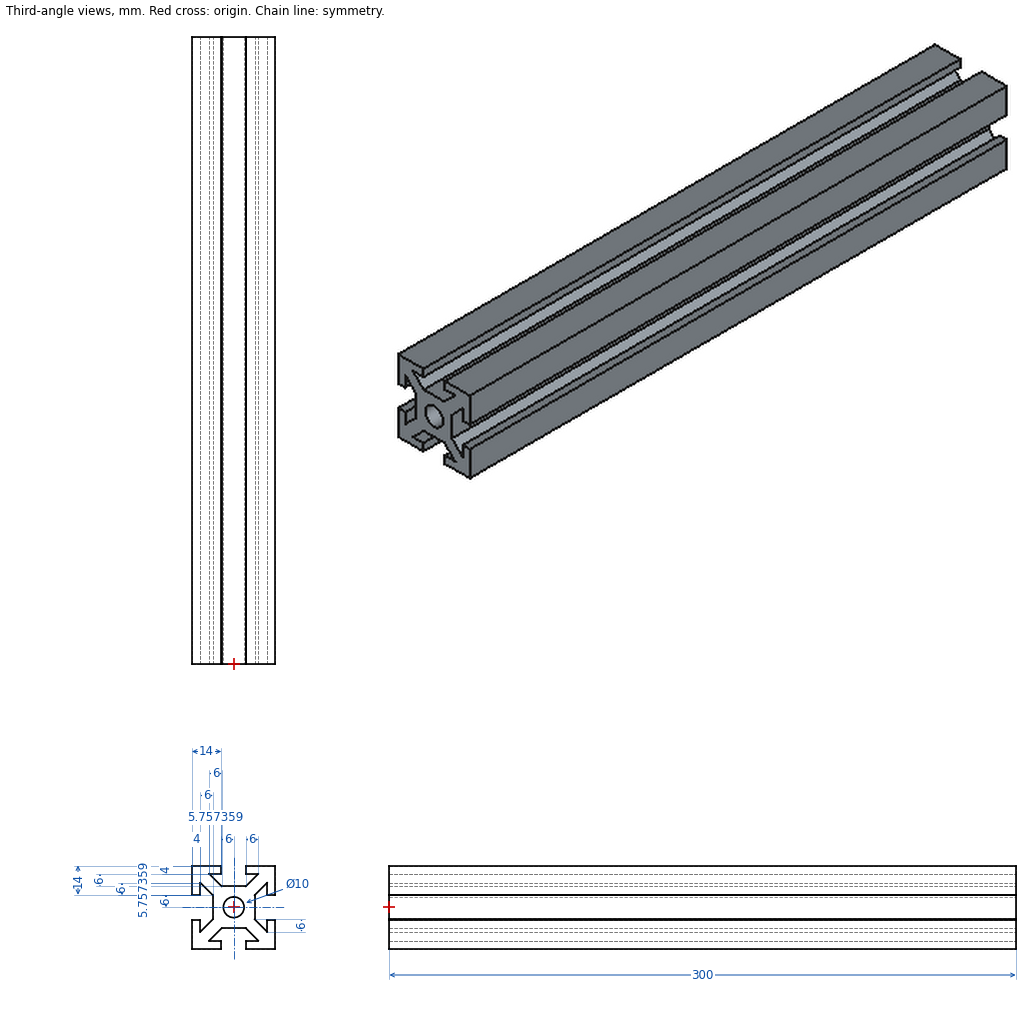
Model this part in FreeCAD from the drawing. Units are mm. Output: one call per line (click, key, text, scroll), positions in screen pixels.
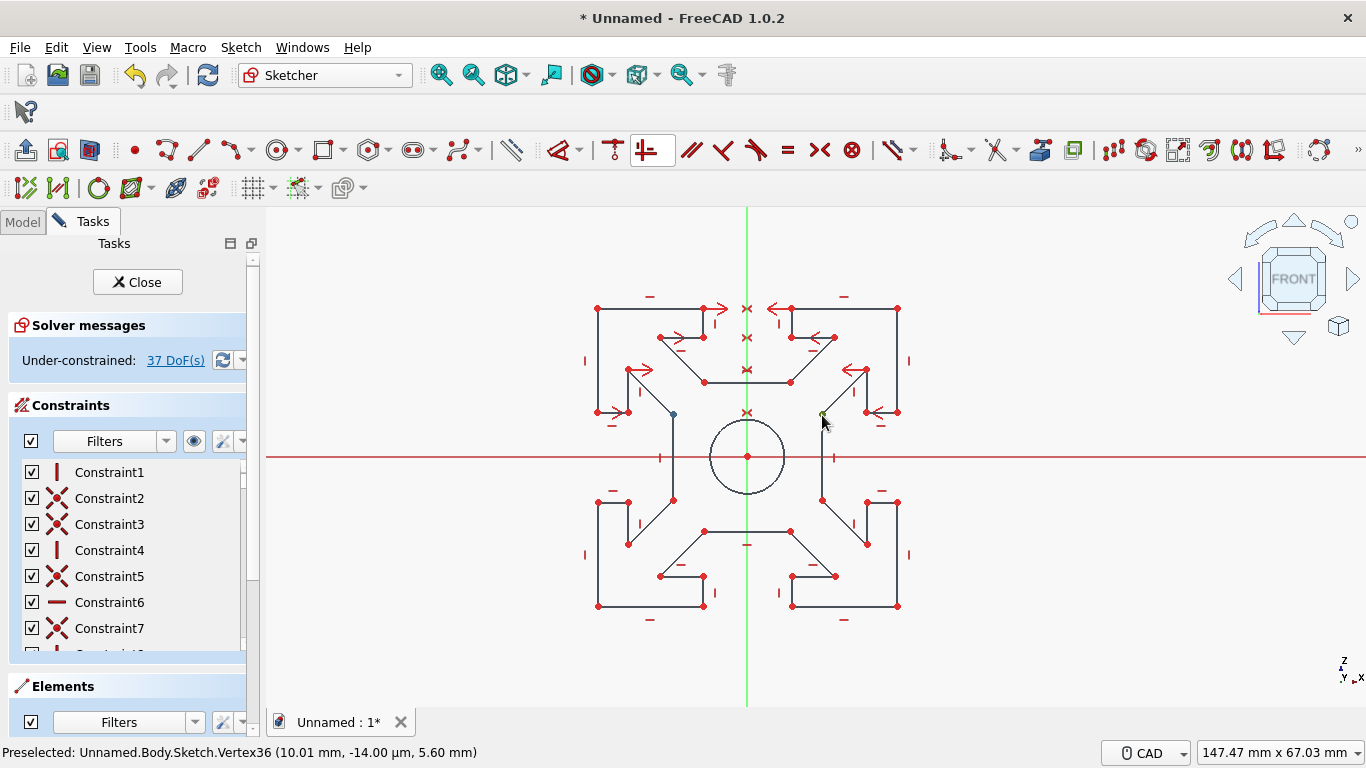
click(747, 647)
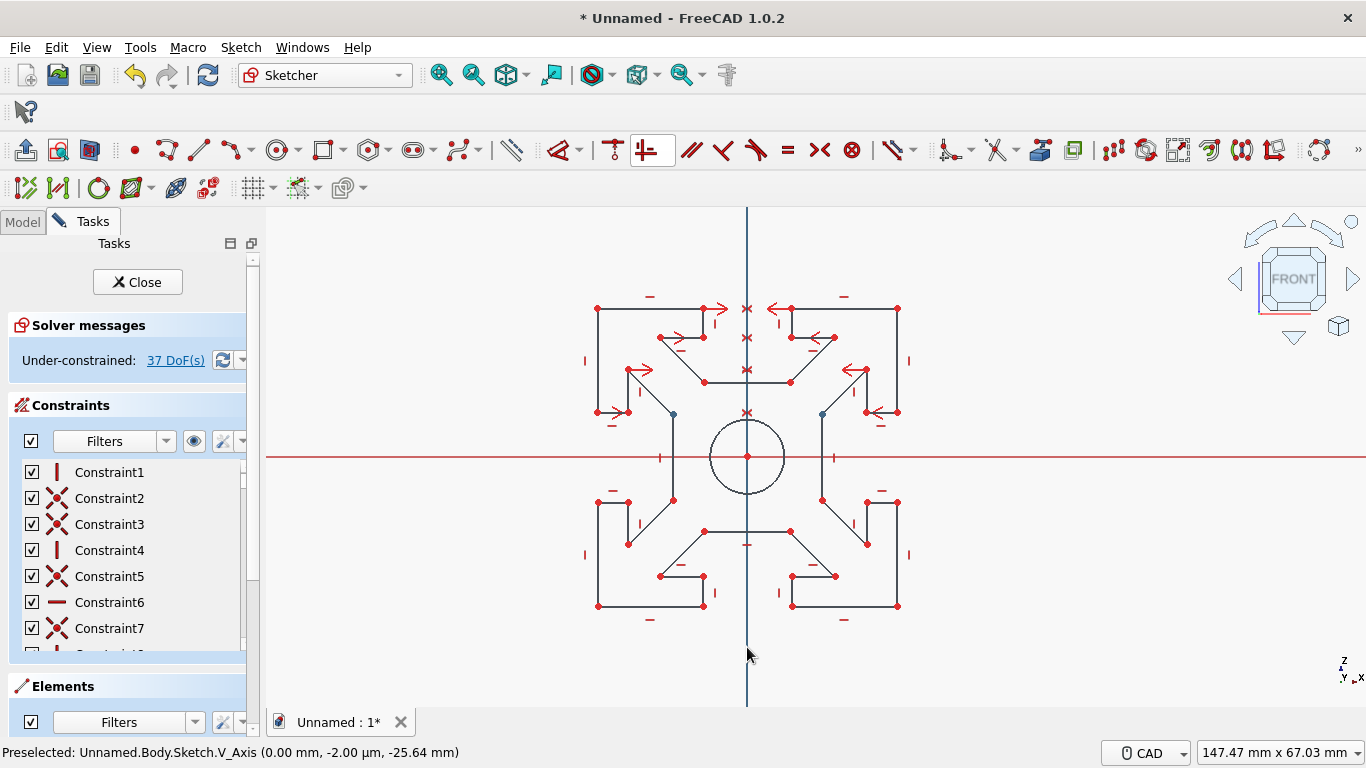
key(s)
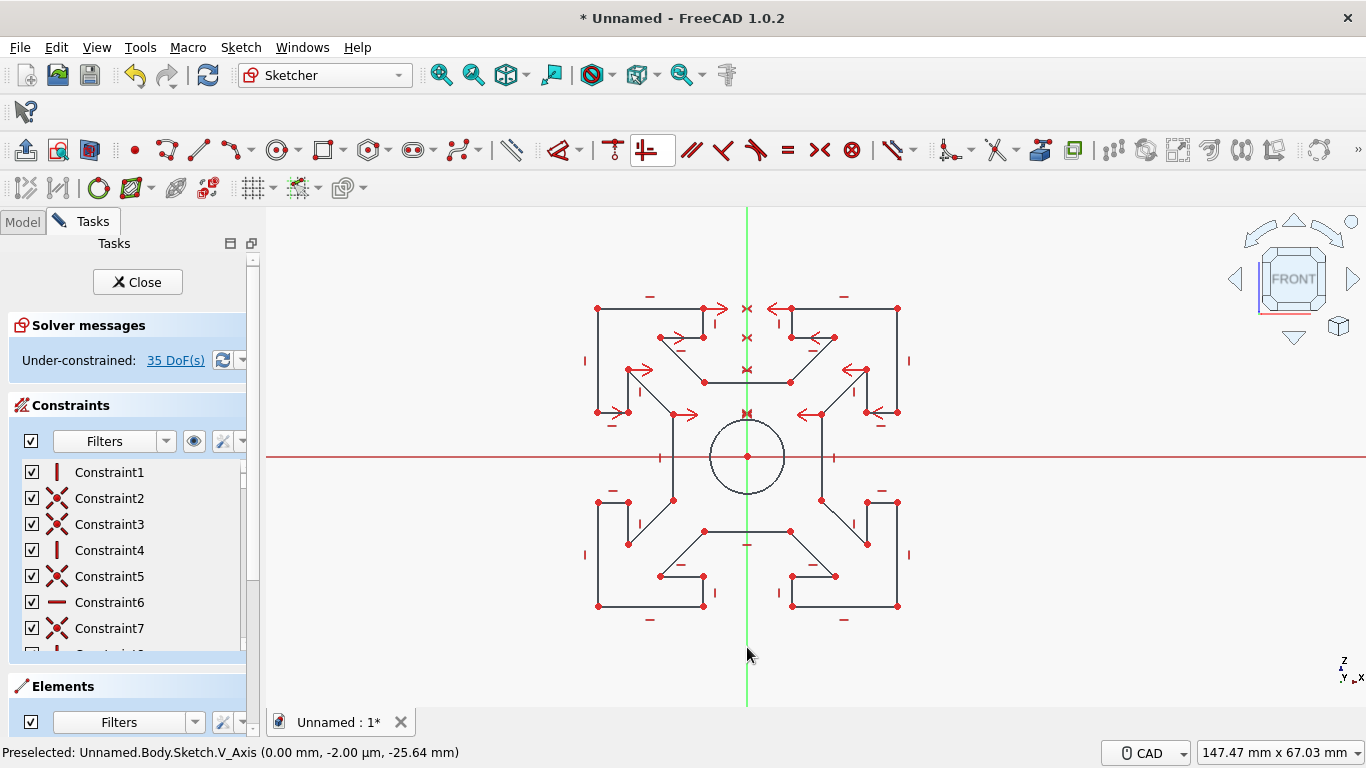
click(867, 370)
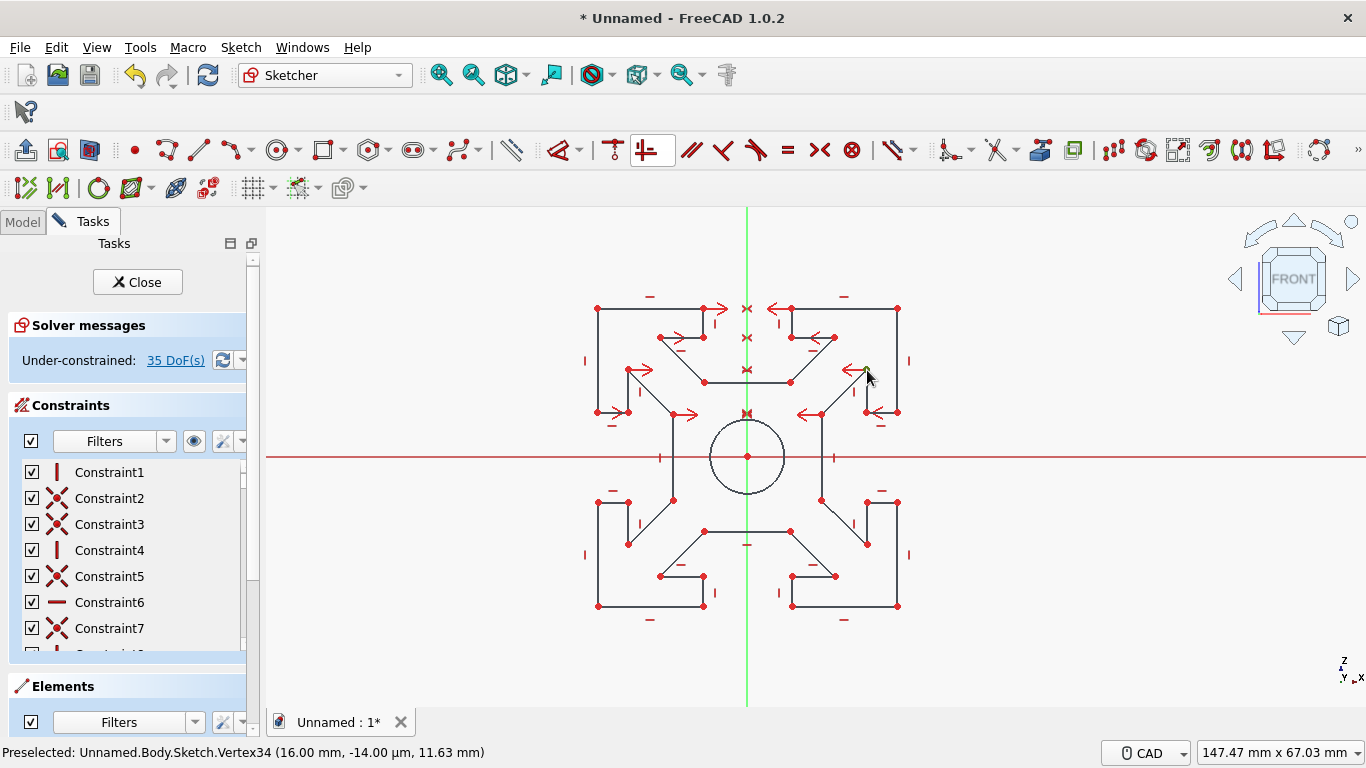
click(867, 545)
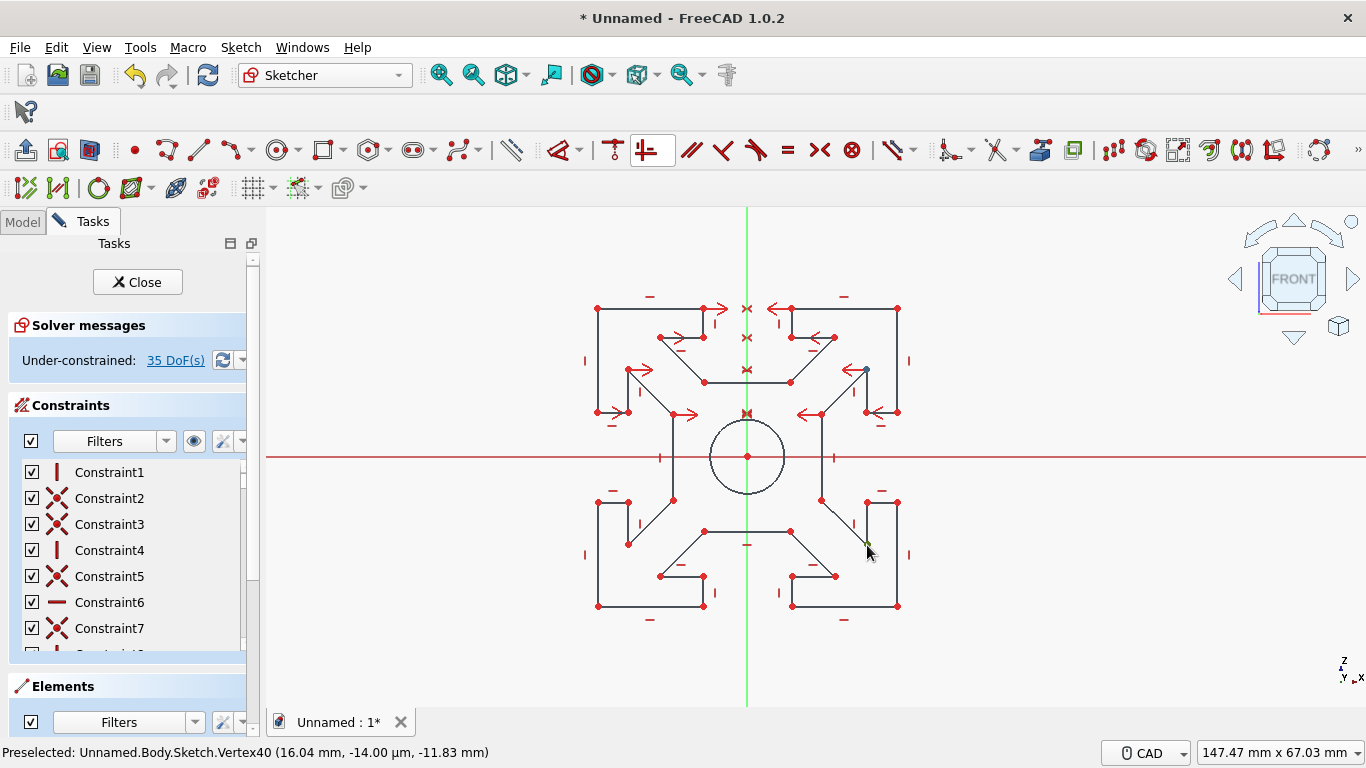
click(359, 457)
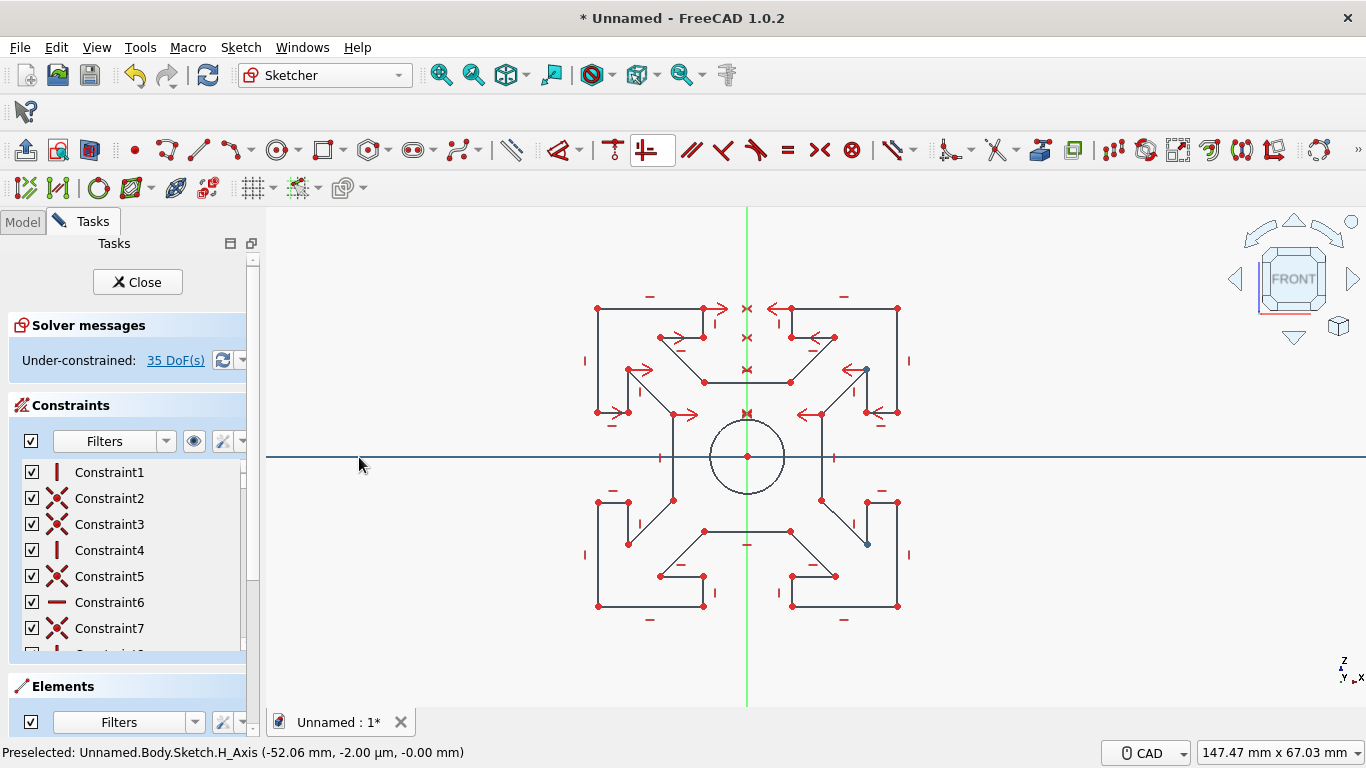
click(820, 150)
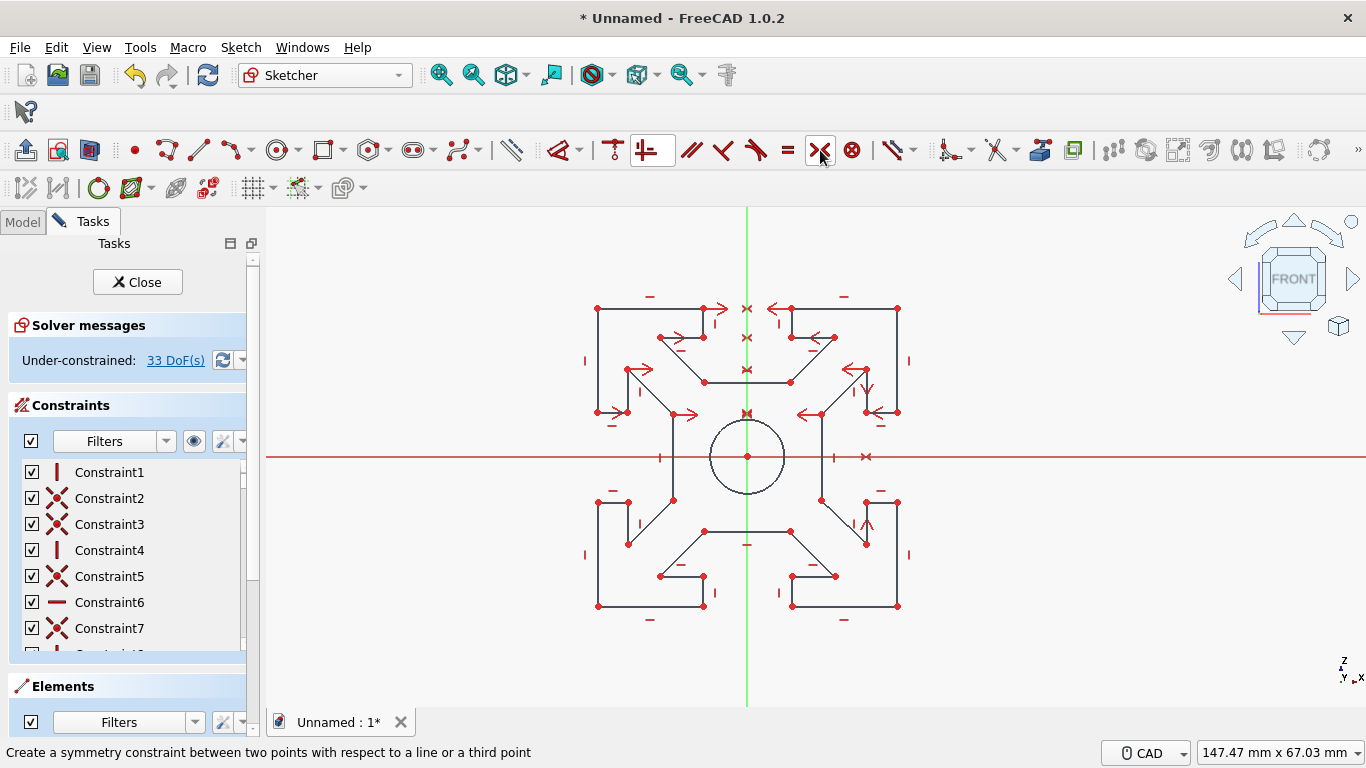
click(897, 413)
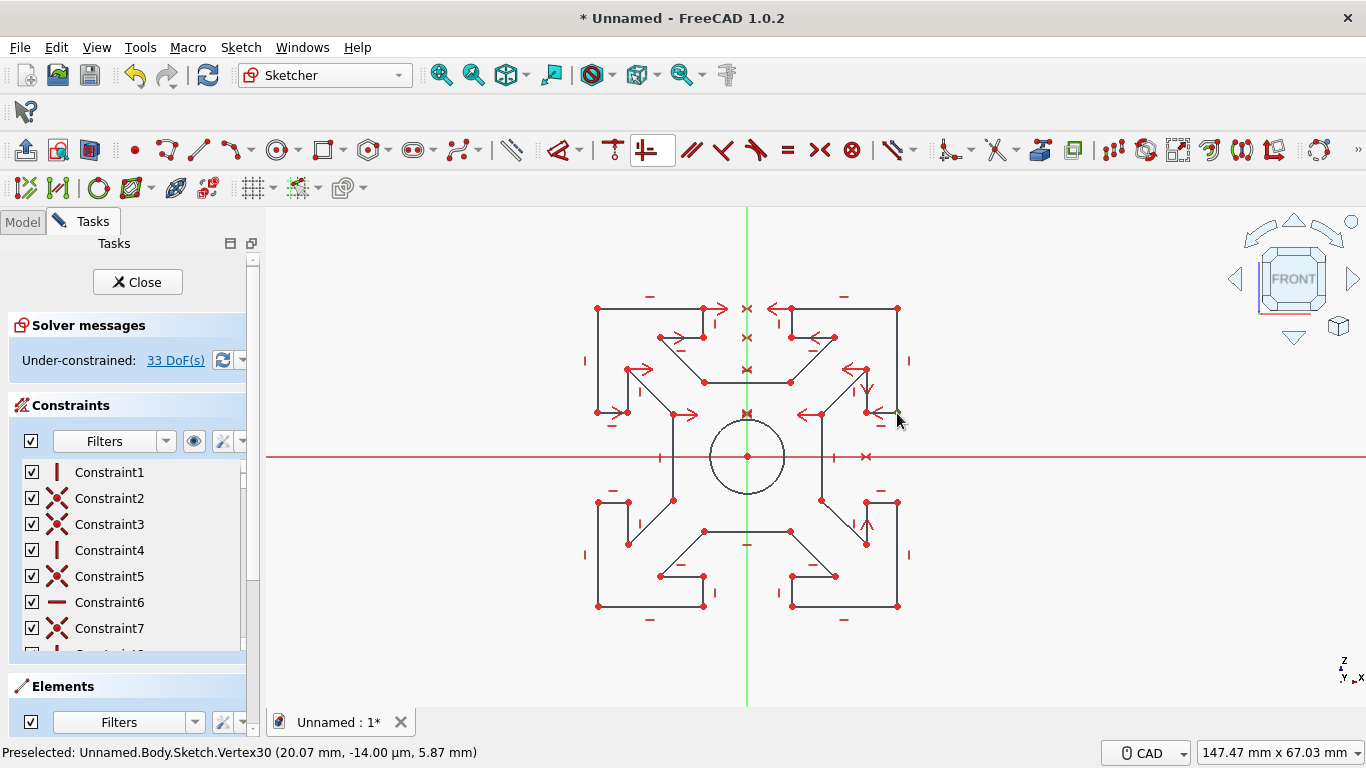
click(897, 503)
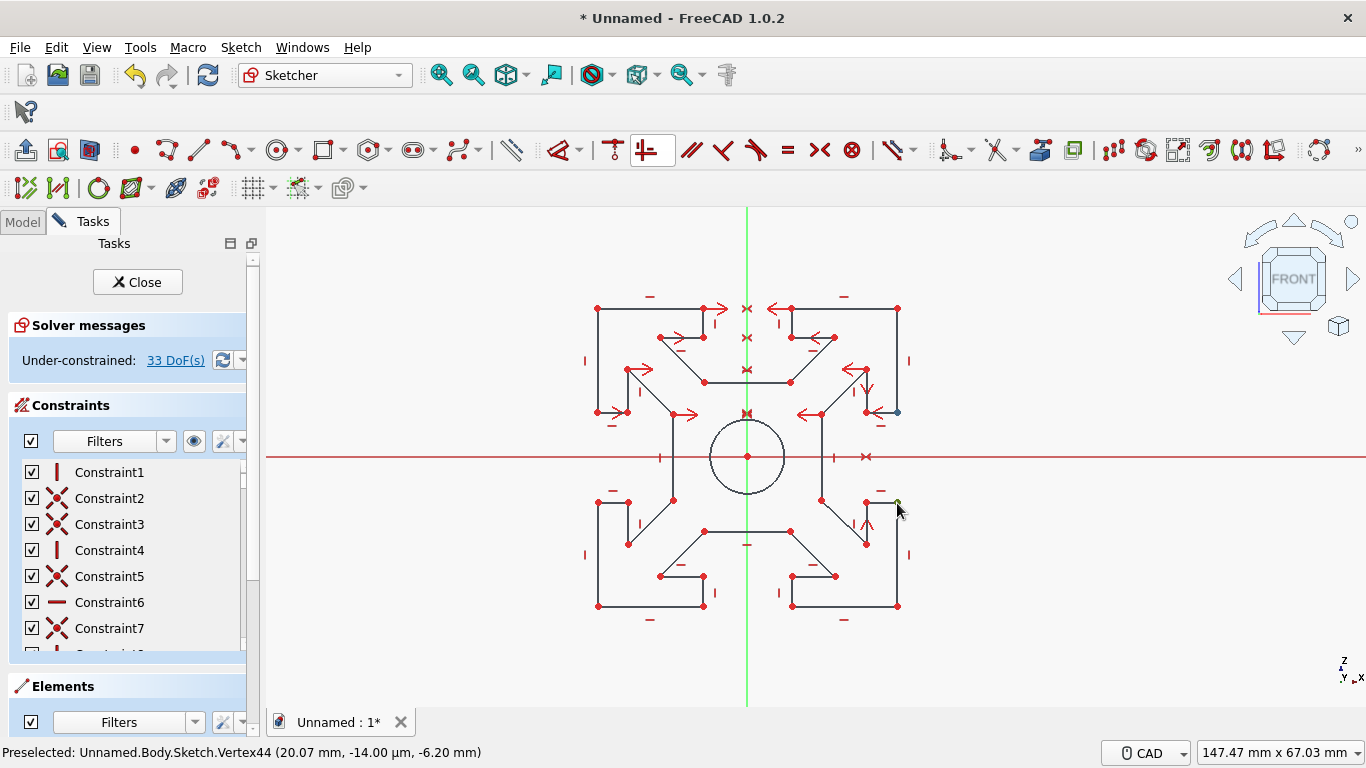
click(359, 457)